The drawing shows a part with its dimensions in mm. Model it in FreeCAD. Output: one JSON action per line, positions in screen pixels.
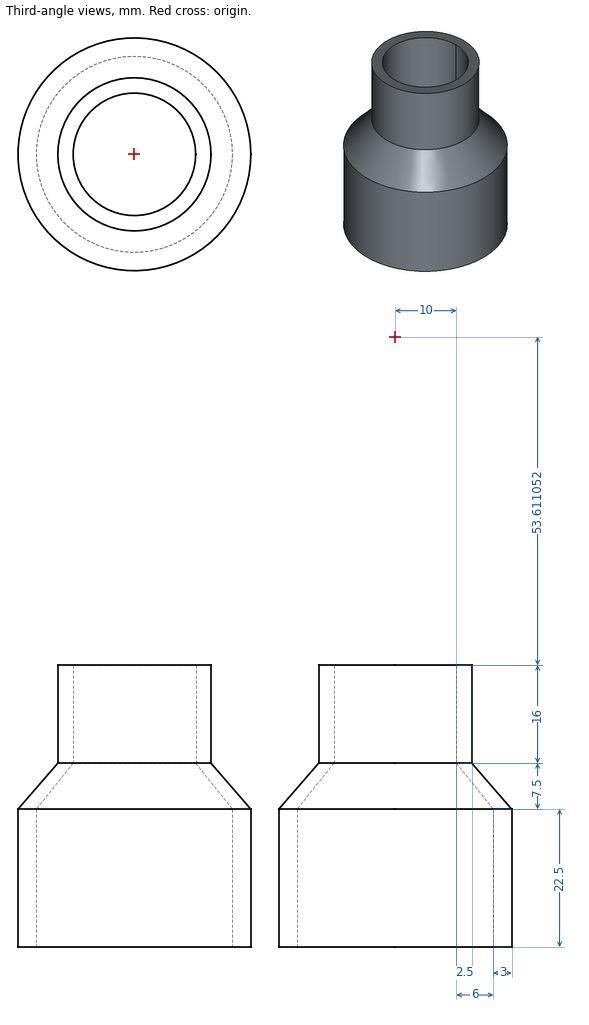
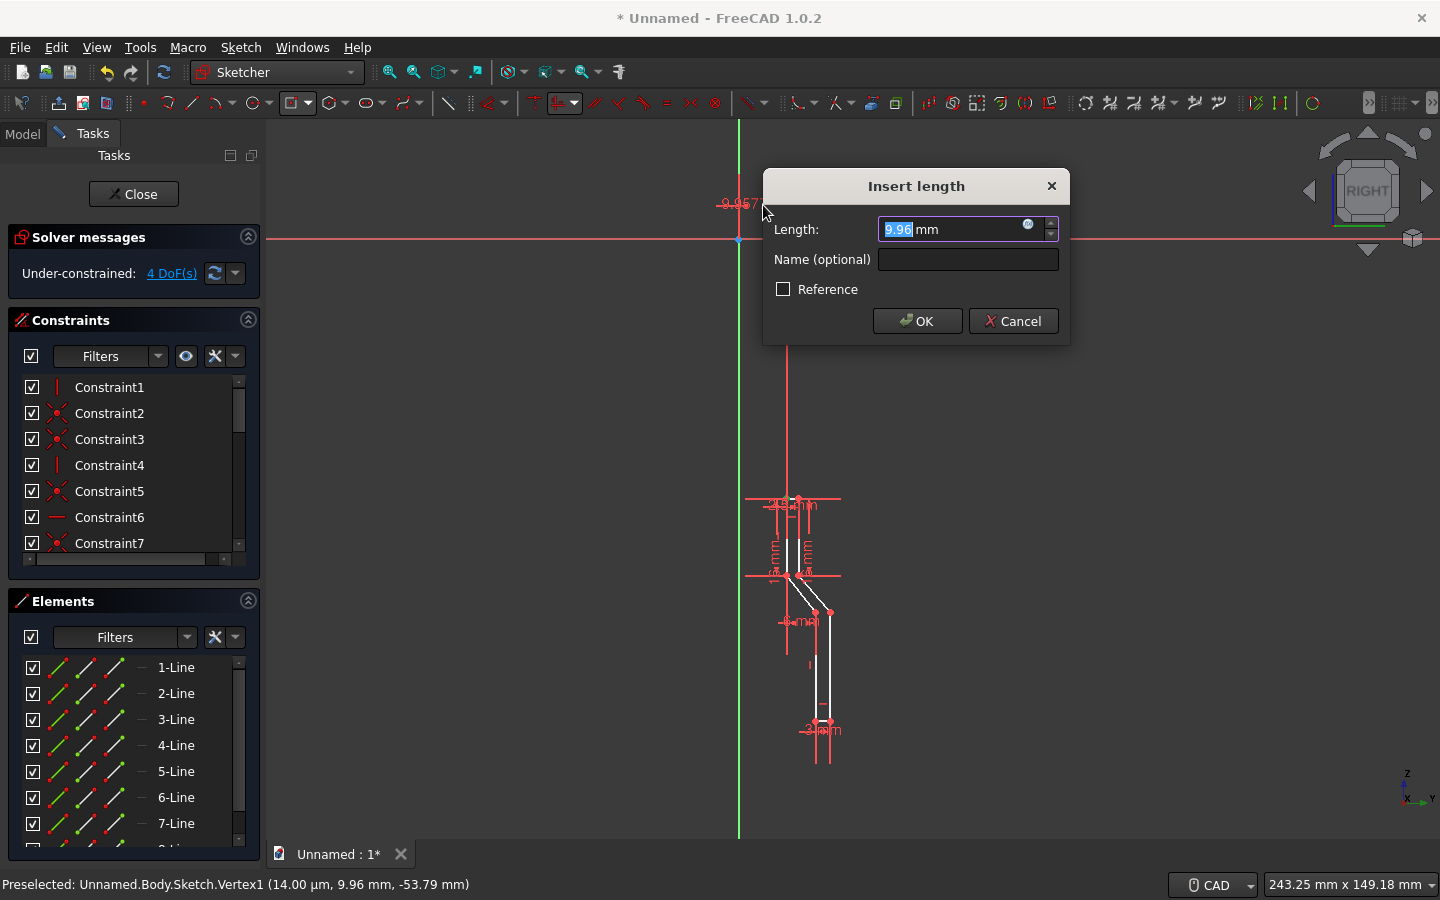
{"action": "type", "text": "10"}
{"action": "key", "text": "Return"}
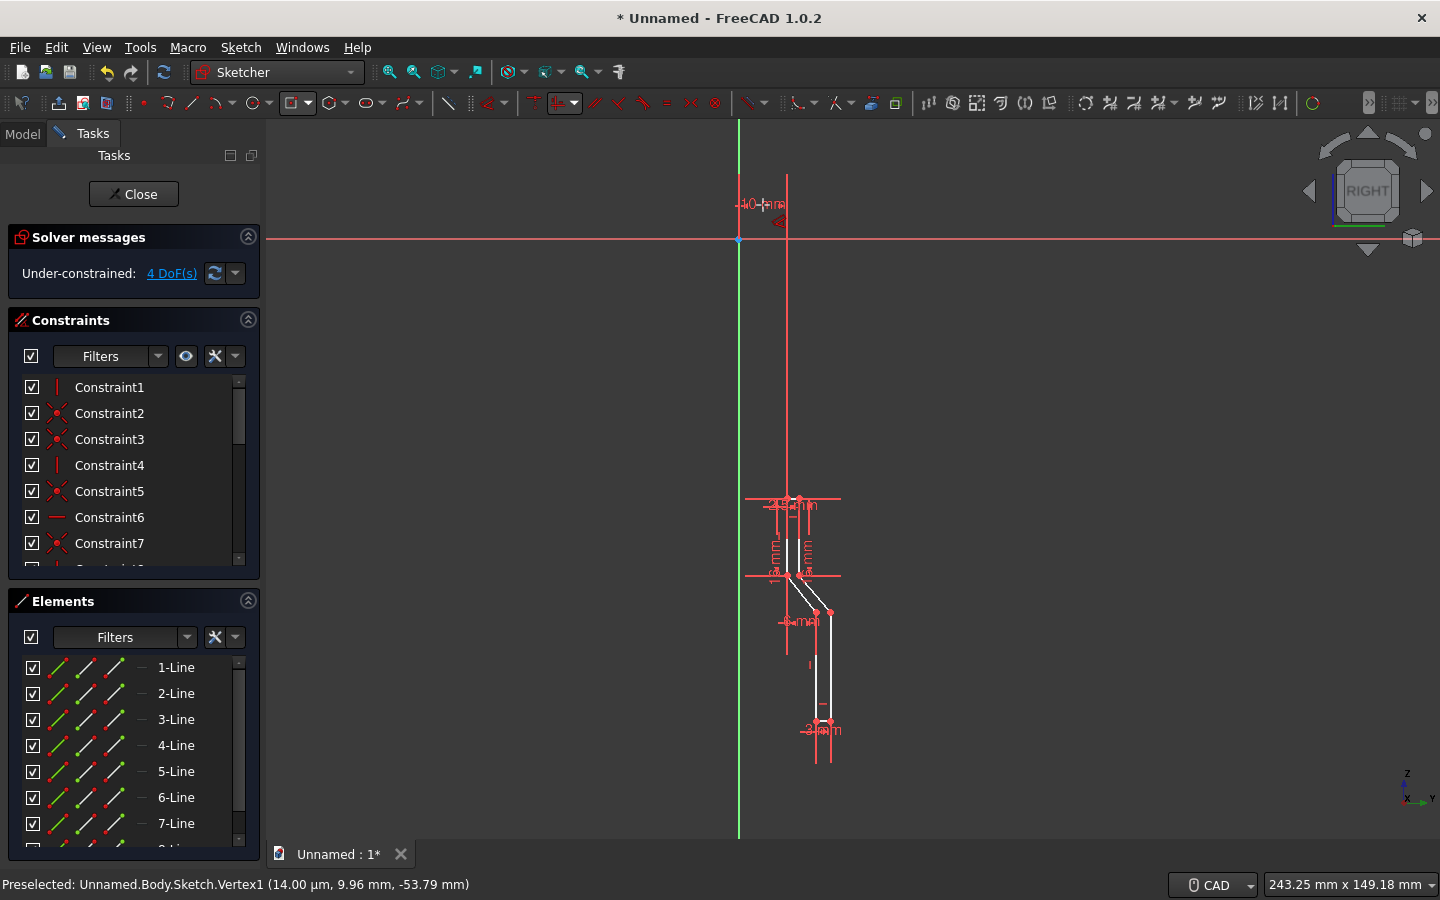
{"action": "left_click", "coordinate": [816, 645]}
{"action": "left_click", "coordinate": [850, 667]}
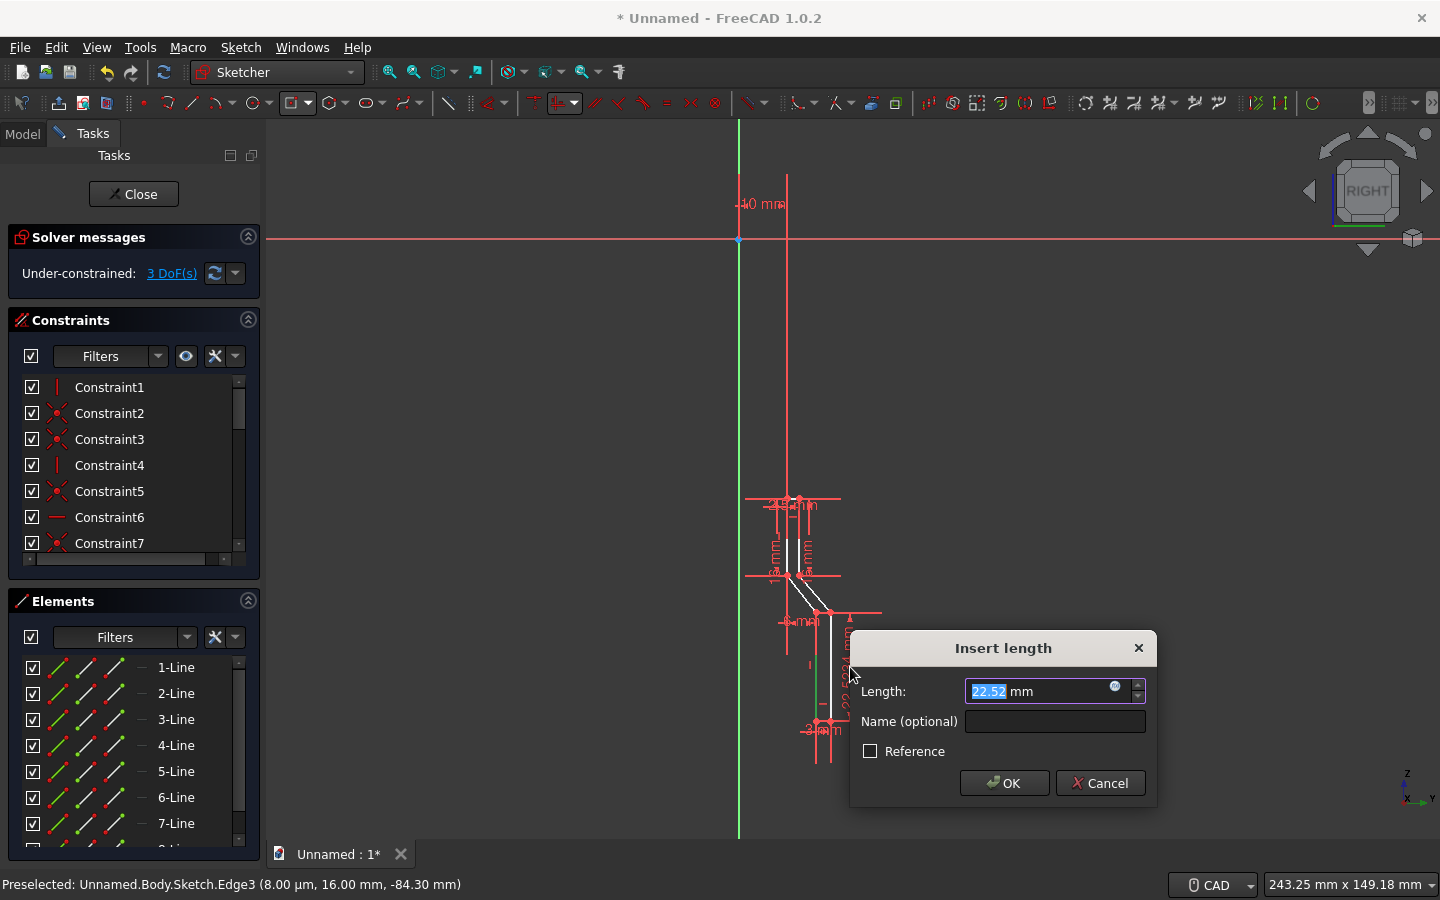
{"action": "type", "text": "22.5"}
{"action": "key", "text": "Return"}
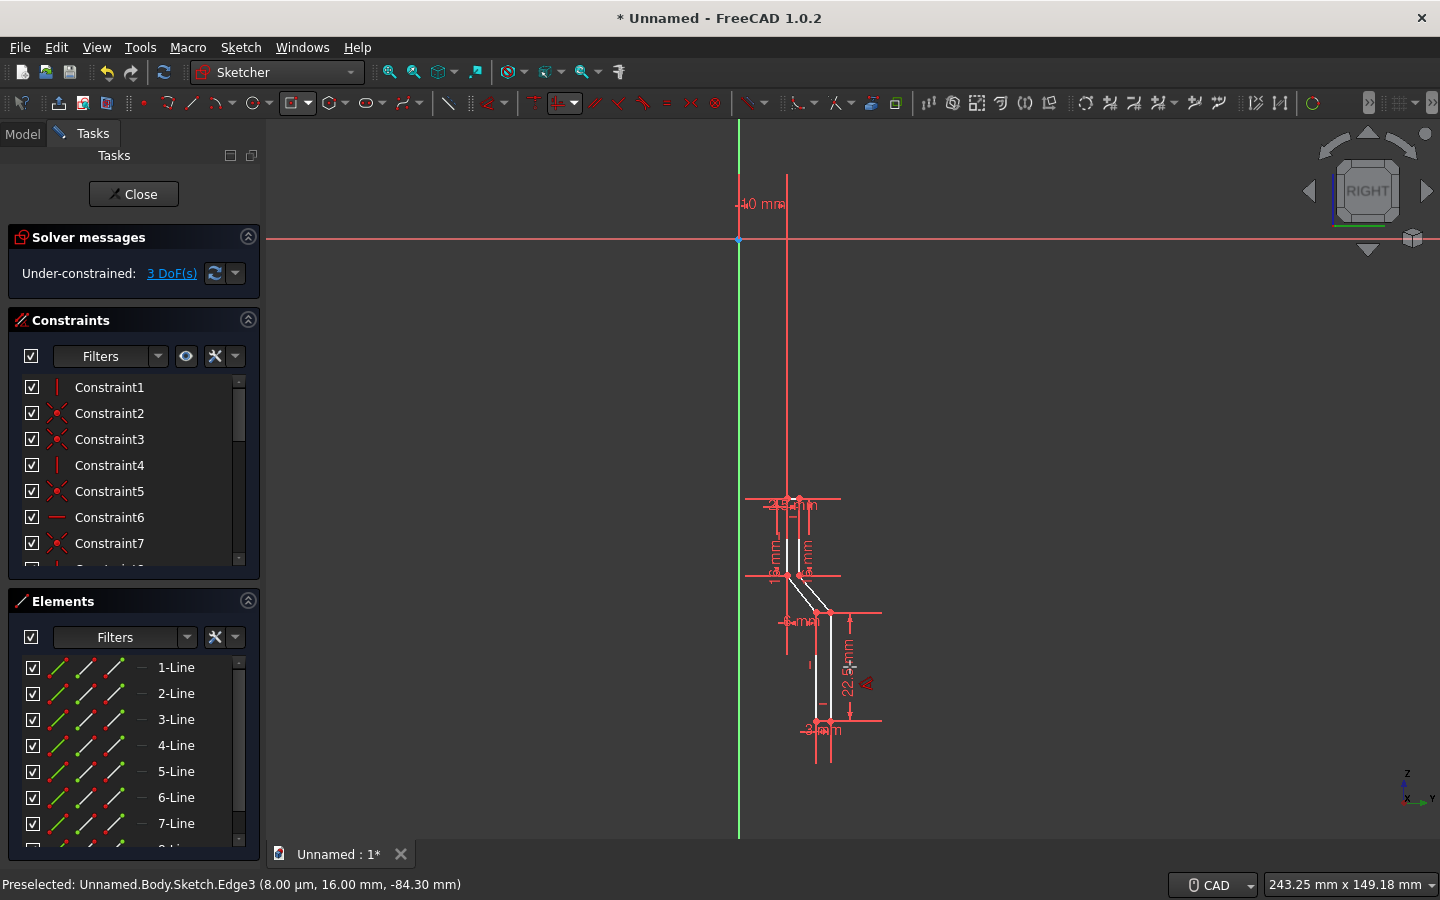
{"action": "left_click", "coordinate": [831, 689]}
{"action": "left_click", "coordinate": [865, 692]}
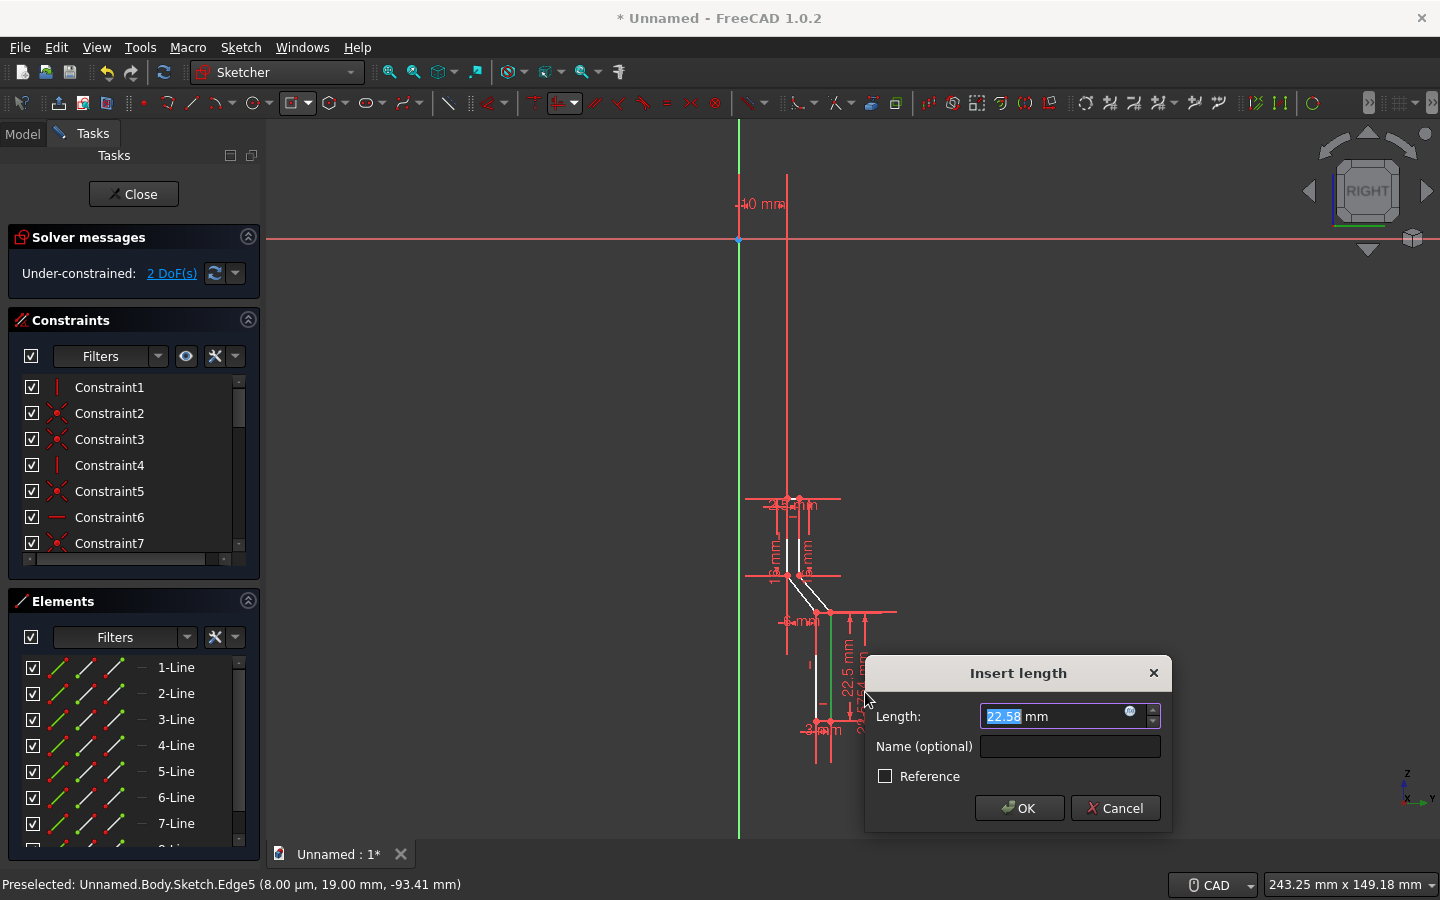
{"action": "type", "text": "22.5"}
{"action": "key", "text": "Return"}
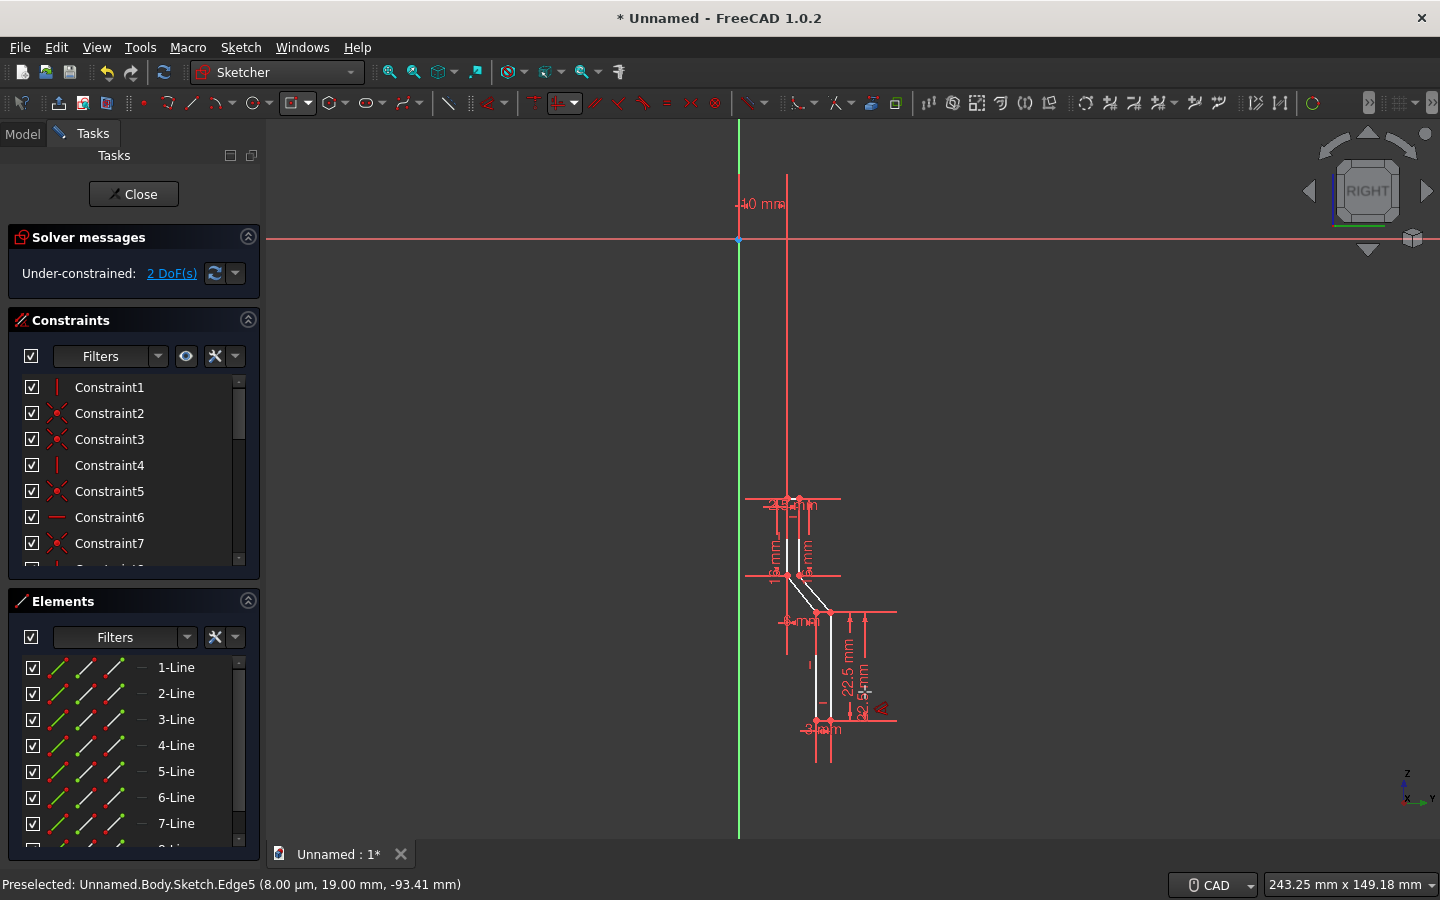
{"action": "scroll", "coordinate": [796, 587], "scroll_direction": "up", "scroll_amount": 2}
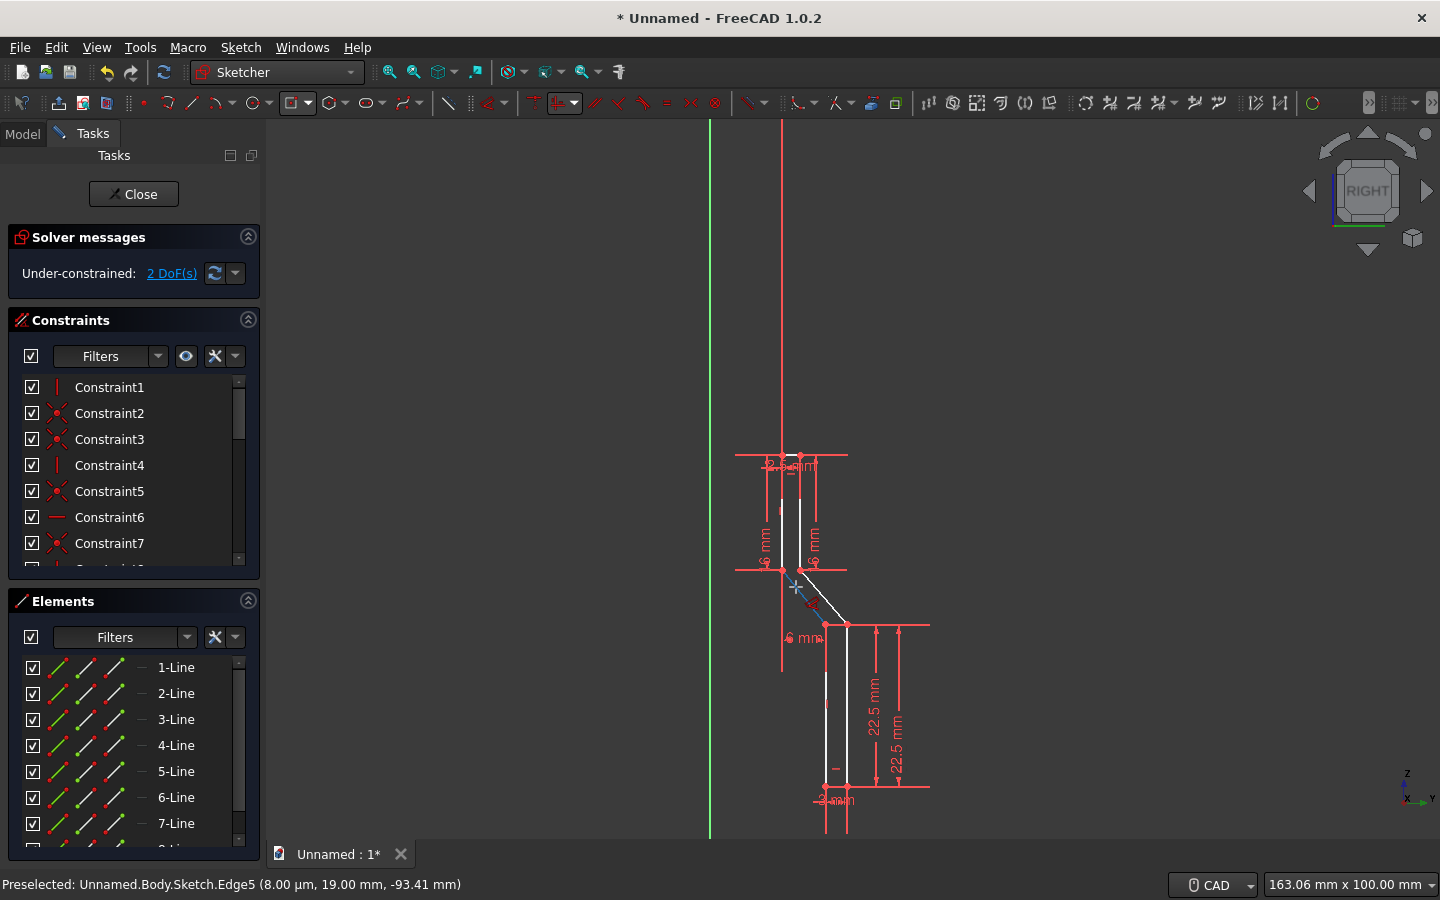
{"action": "left_click", "coordinate": [795, 587]}
{"action": "left_click", "coordinate": [860, 597]}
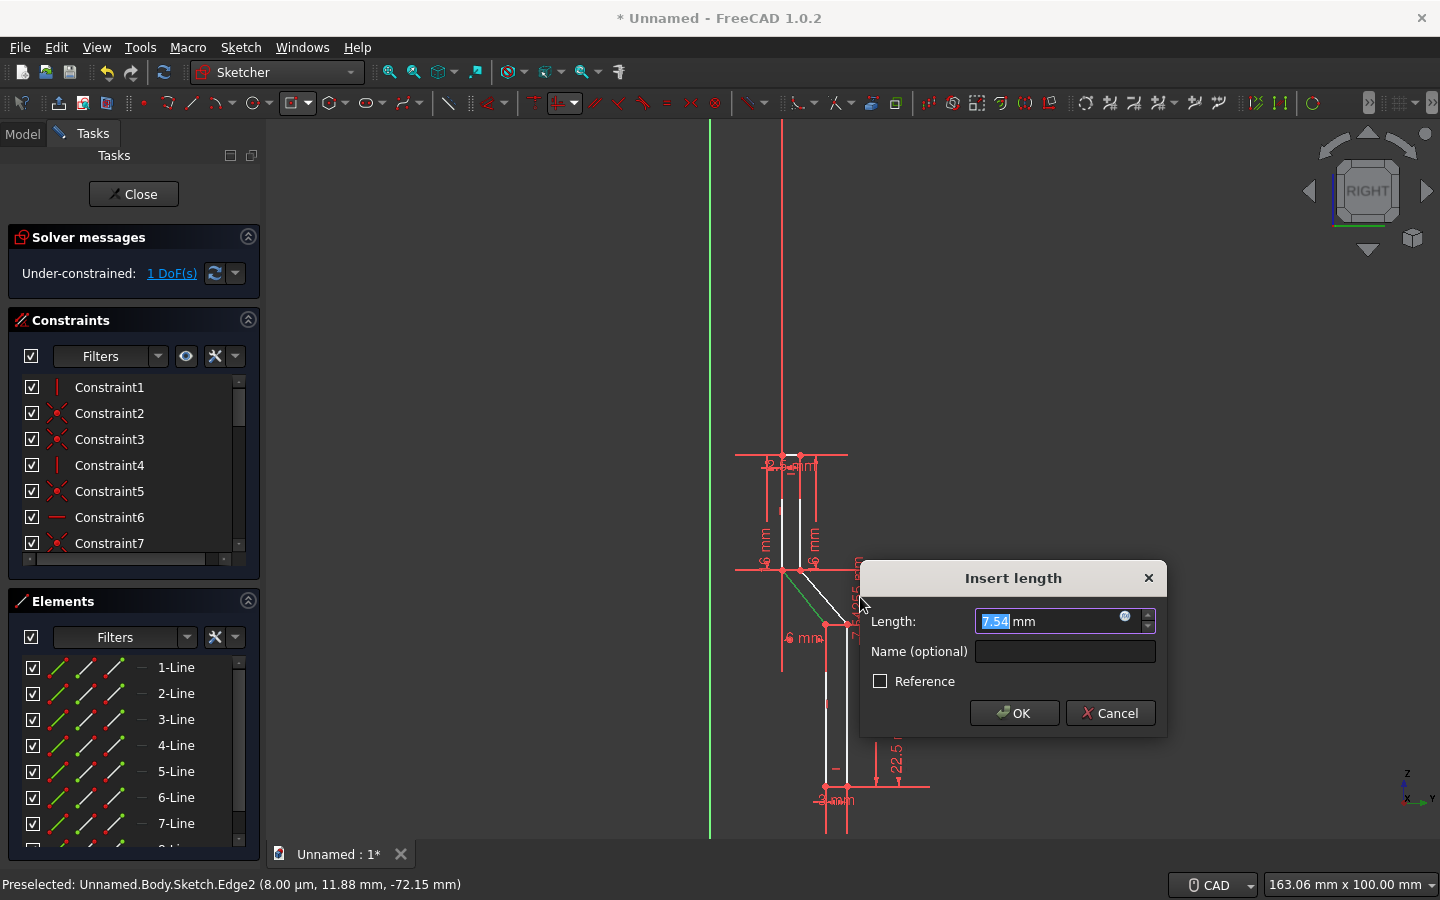
{"action": "type", "text": "7.5"}
{"action": "key", "text": "Return"}